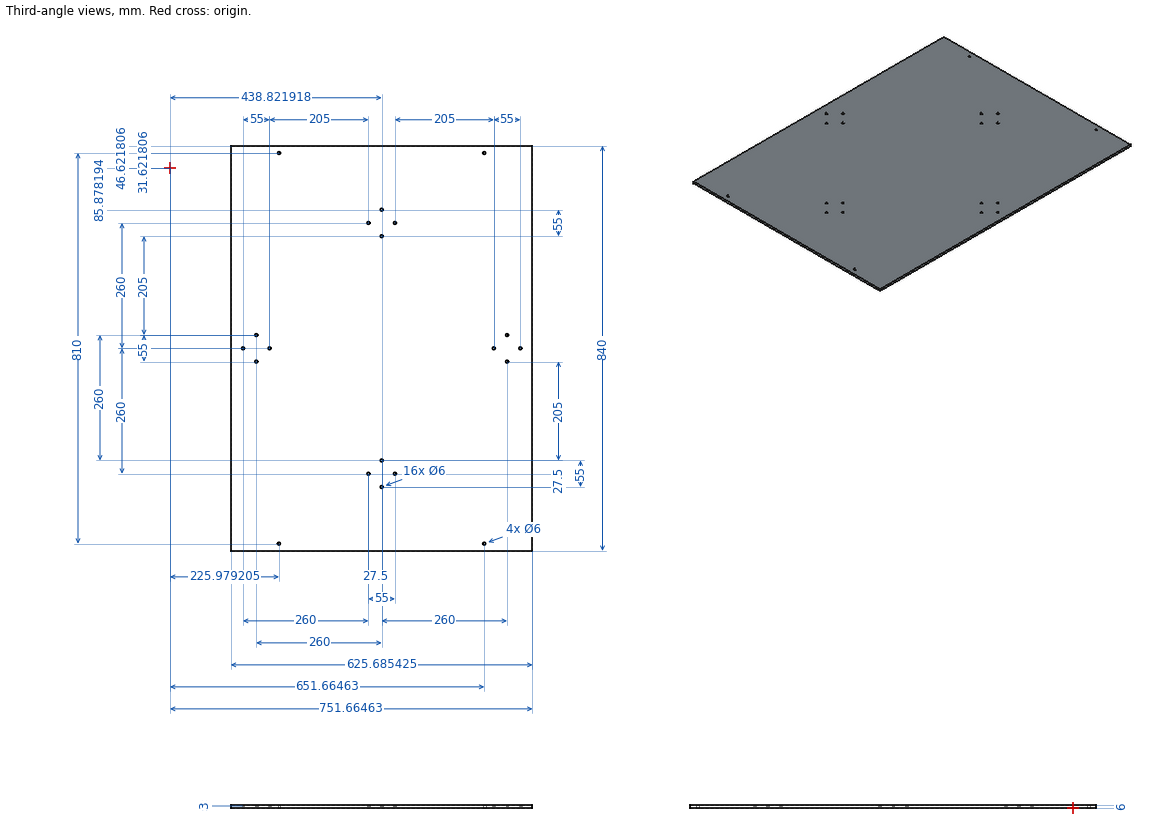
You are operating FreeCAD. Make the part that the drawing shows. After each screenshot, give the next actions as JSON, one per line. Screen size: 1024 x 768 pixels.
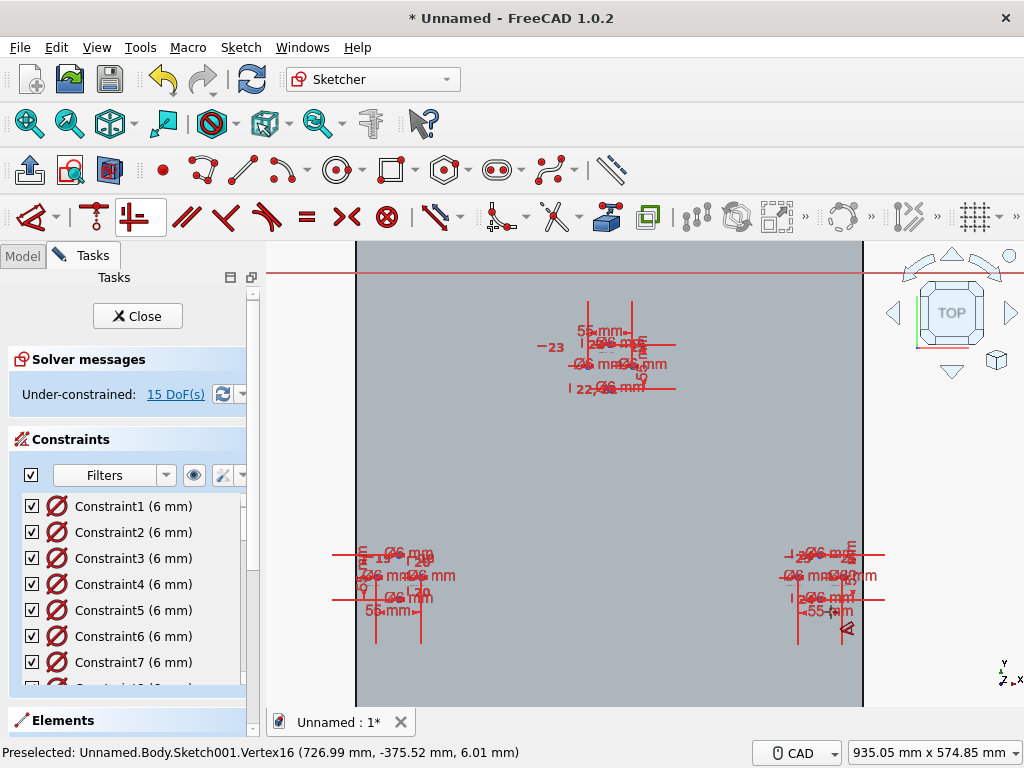
{"action": "scroll", "coordinate": [610, 391], "scroll_direction": "down", "scroll_amount": 3}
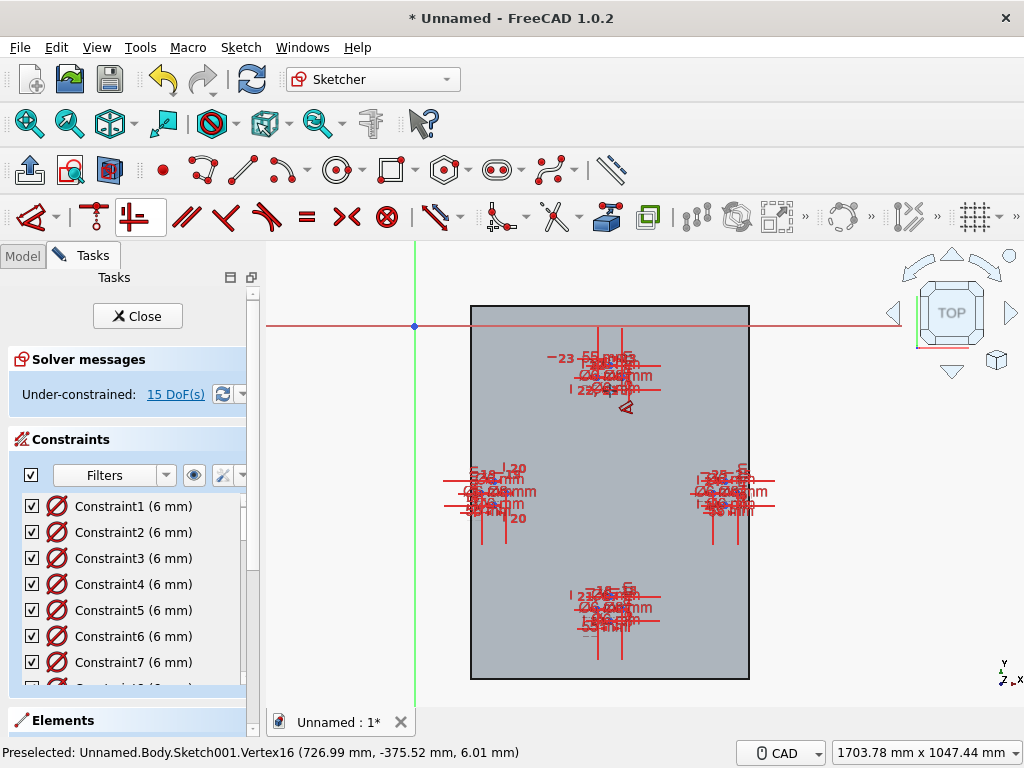
{"action": "left_click", "coordinate": [598, 610]}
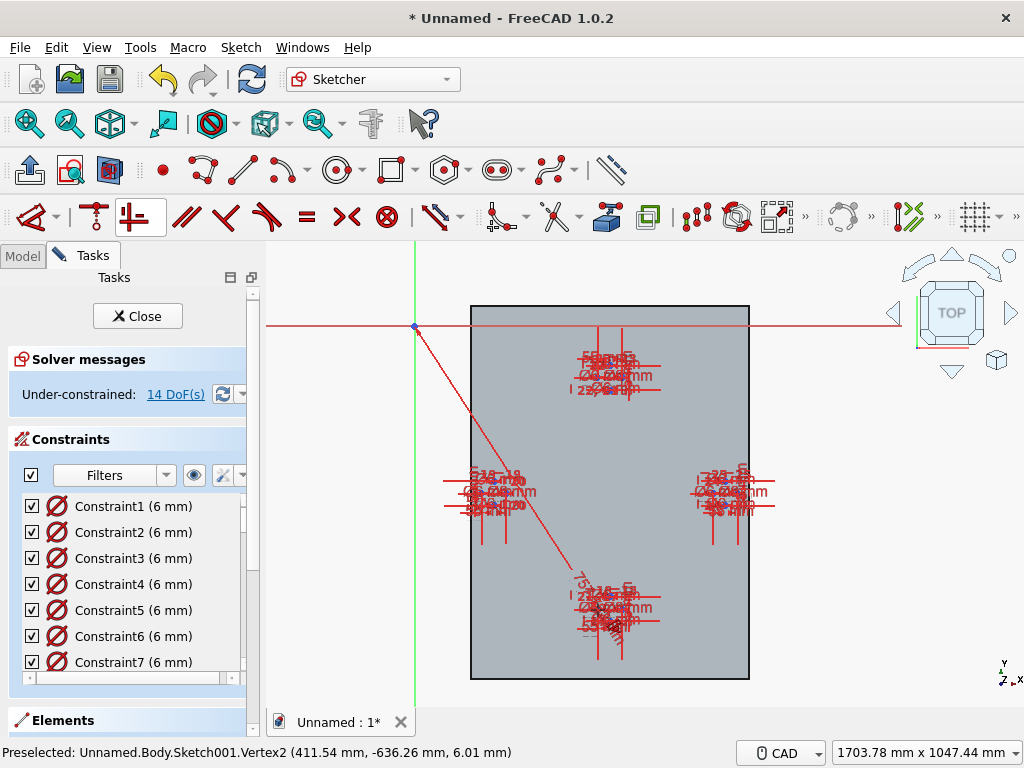
{"action": "left_click", "coordinate": [482, 494]}
{"action": "left_click", "coordinate": [513, 644]}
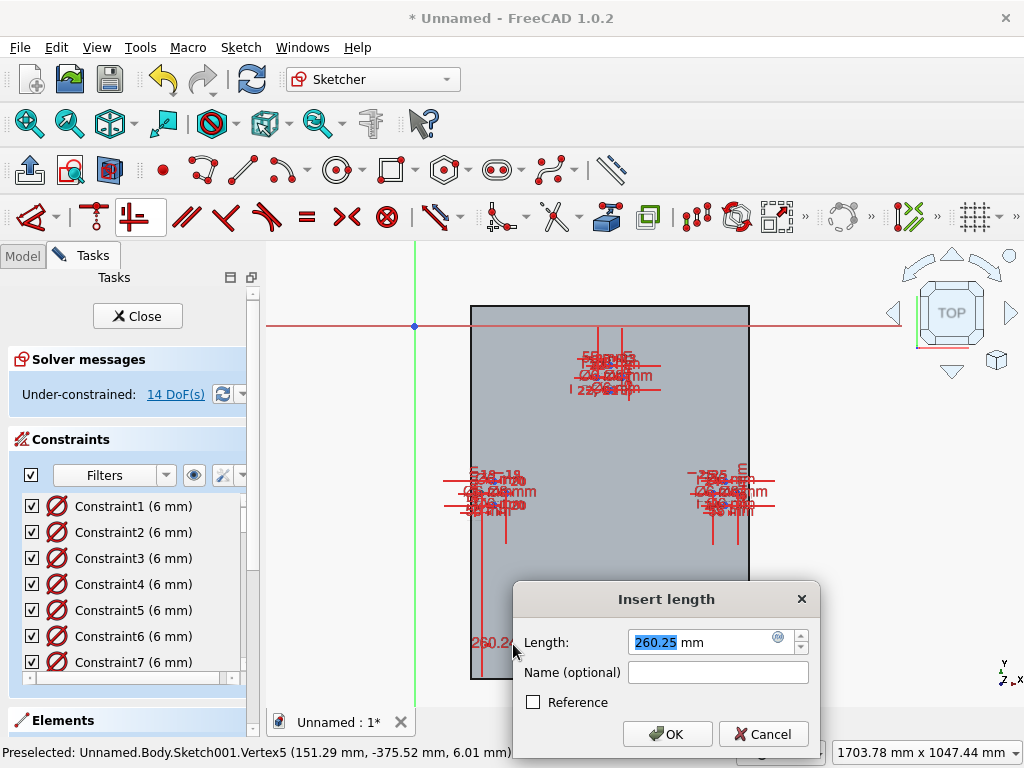
{"action": "type", "text": "260"}
{"action": "key", "text": "Return"}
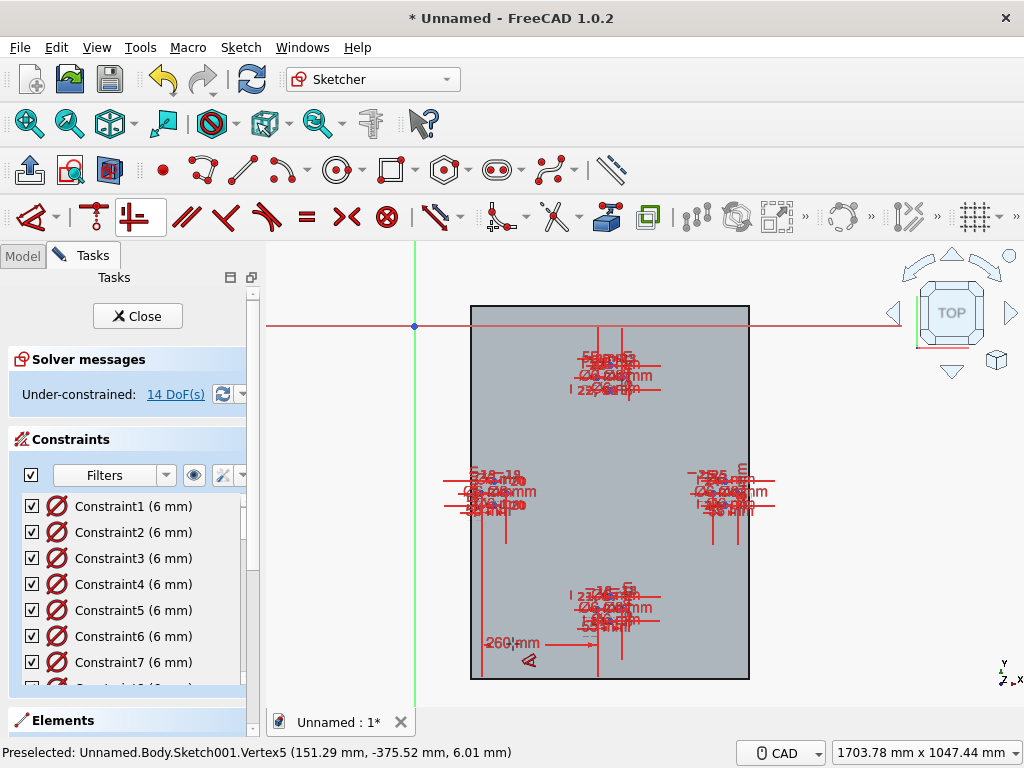
{"action": "left_click", "coordinate": [598, 610]}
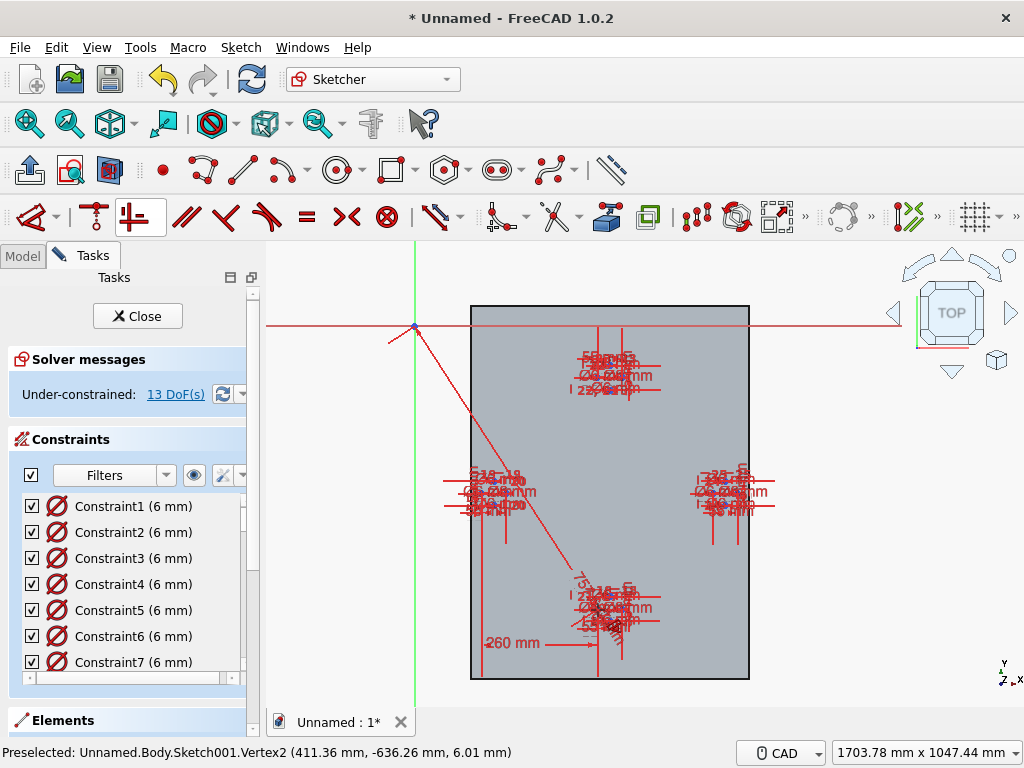
{"action": "left_click", "coordinate": [482, 494]}
{"action": "left_click", "coordinate": [448, 552]}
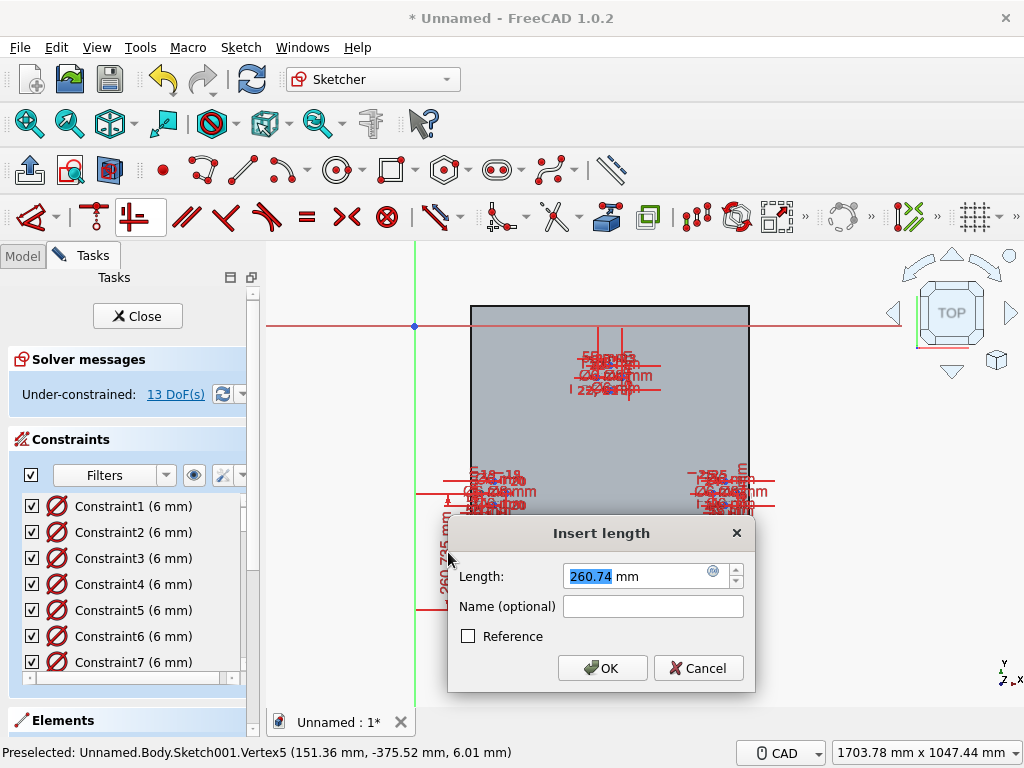
{"action": "type", "text": "260"}
{"action": "key", "text": "Return"}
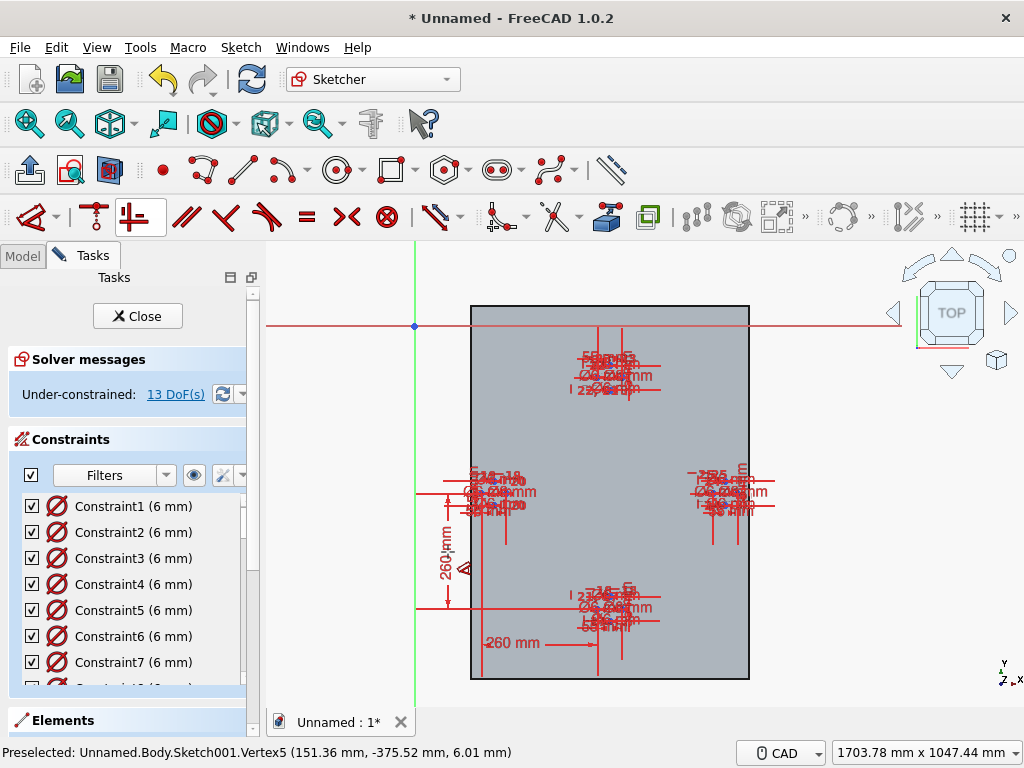
{"action": "left_click", "coordinate": [610, 597]}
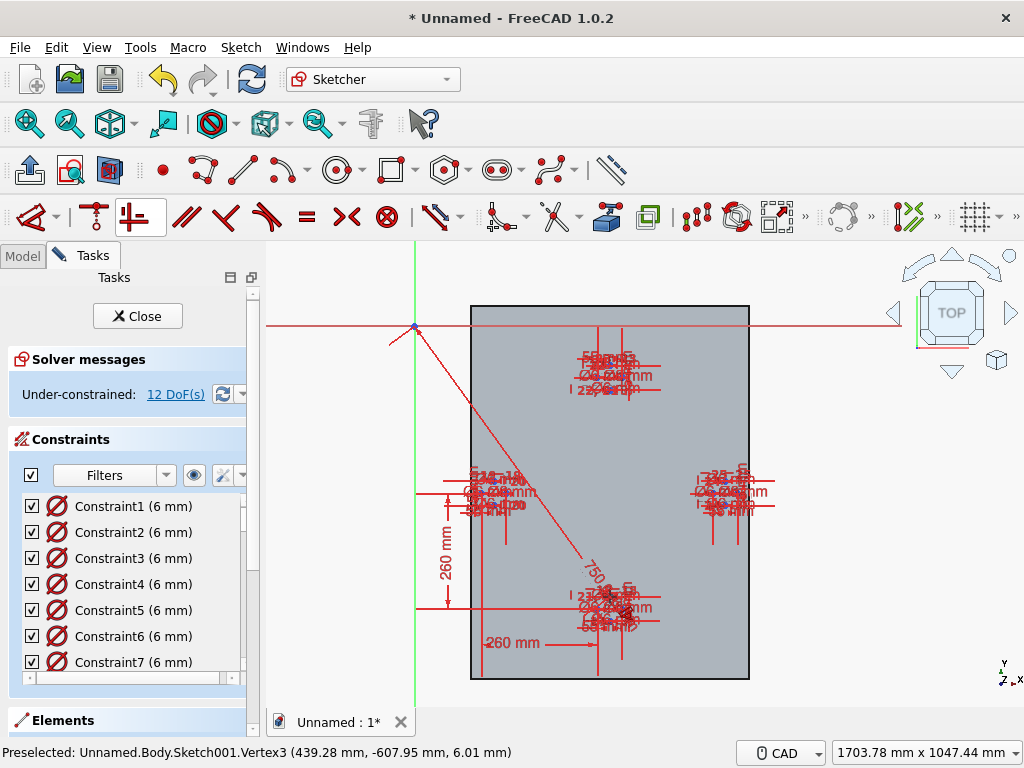
{"action": "left_click", "coordinate": [494, 481]}
{"action": "left_click", "coordinate": [552, 447]}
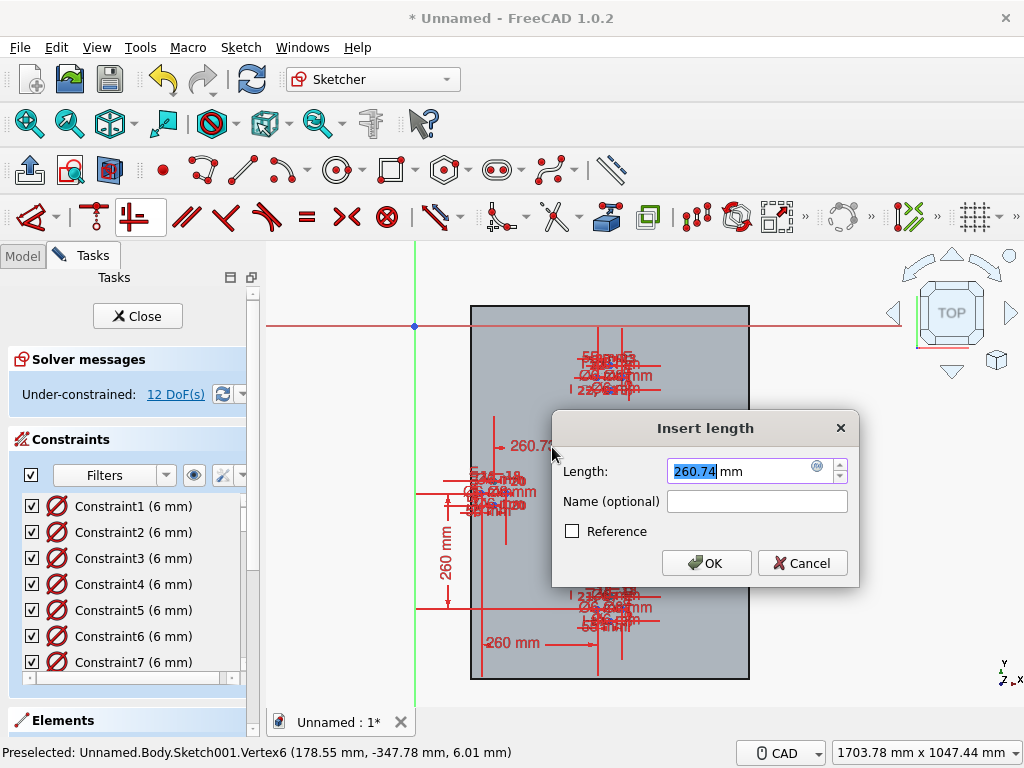
{"action": "type", "text": "260"}
{"action": "key", "text": "Return"}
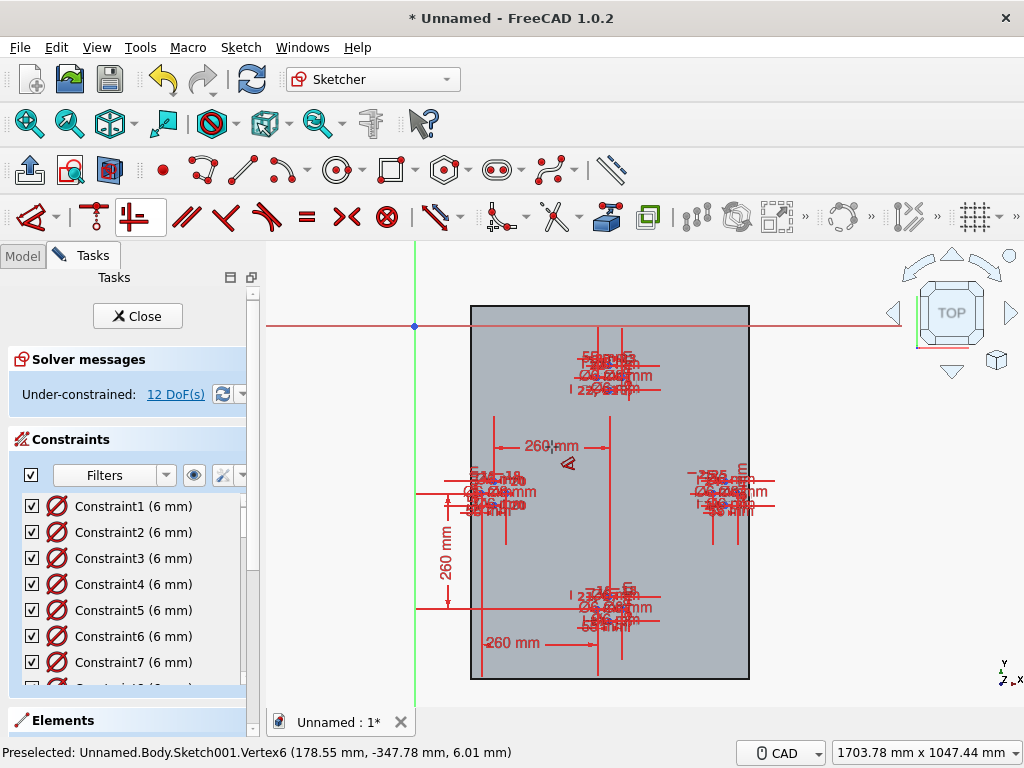
{"action": "left_click", "coordinate": [610, 597]}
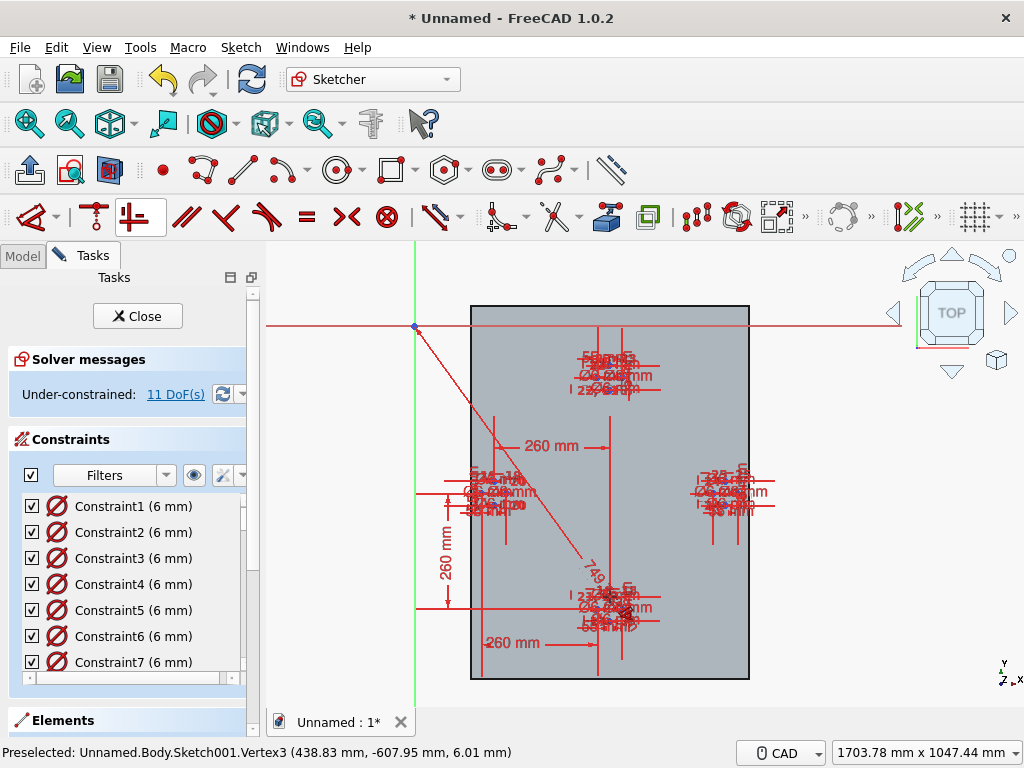
{"action": "left_click", "coordinate": [494, 481]}
{"action": "left_click", "coordinate": [460, 580]}